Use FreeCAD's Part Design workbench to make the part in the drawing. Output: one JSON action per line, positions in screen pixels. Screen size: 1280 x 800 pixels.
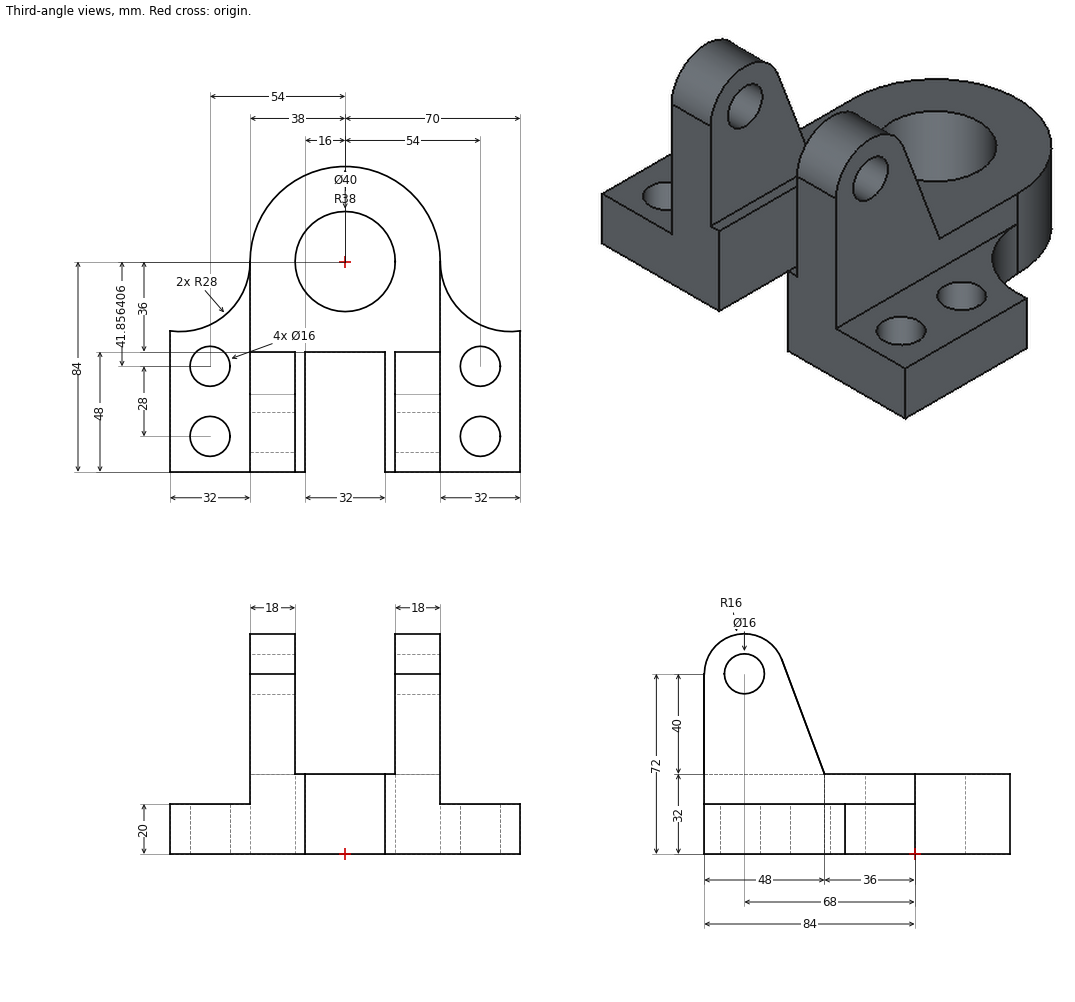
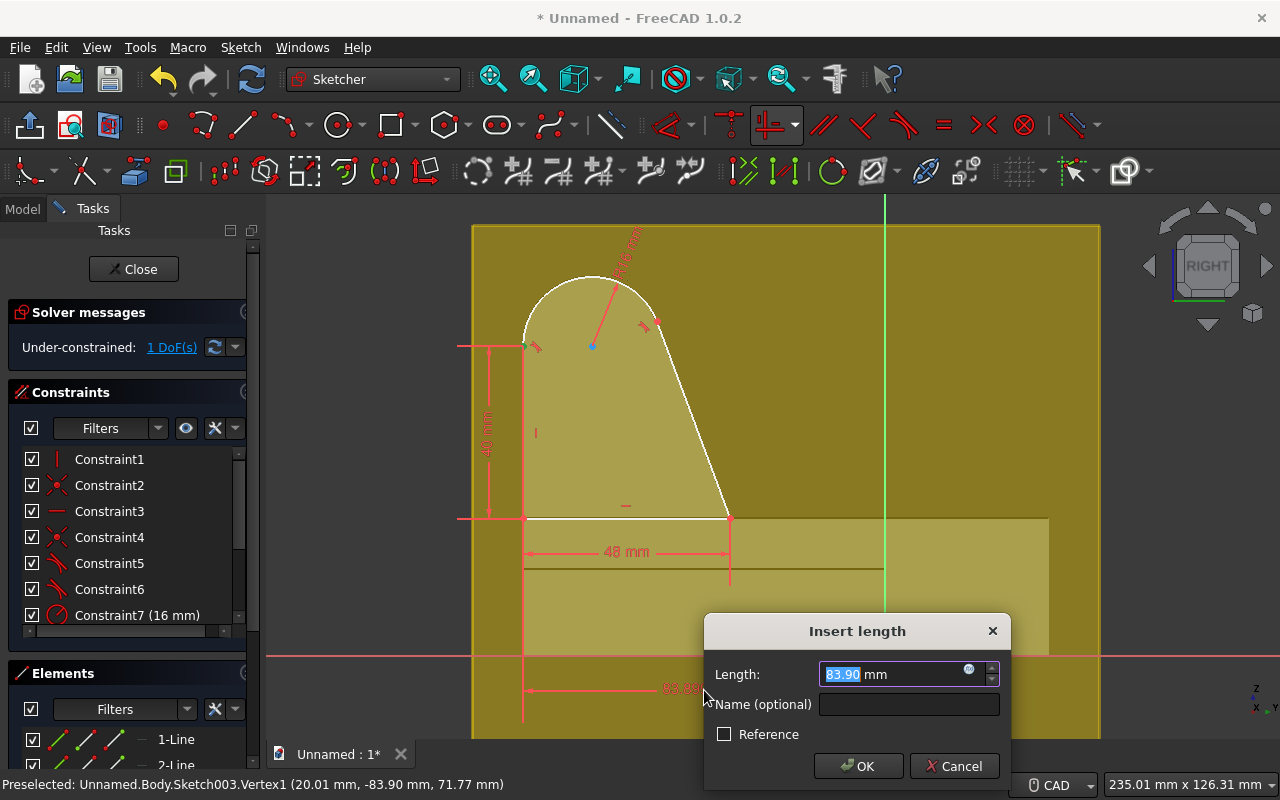
{"action": "type", "text": "84"}
{"action": "key", "text": "Return"}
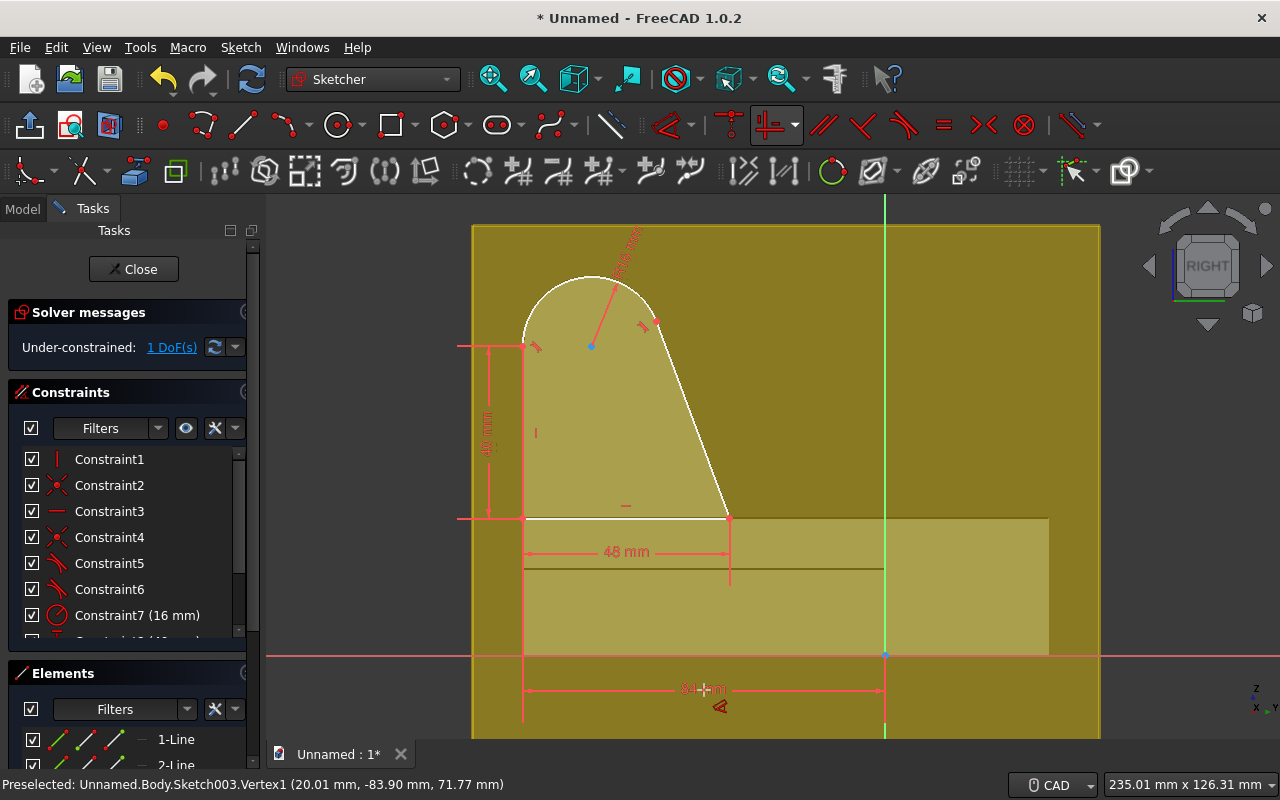
{"action": "left_click", "coordinate": [523, 346]}
{"action": "left_click", "coordinate": [919, 501]}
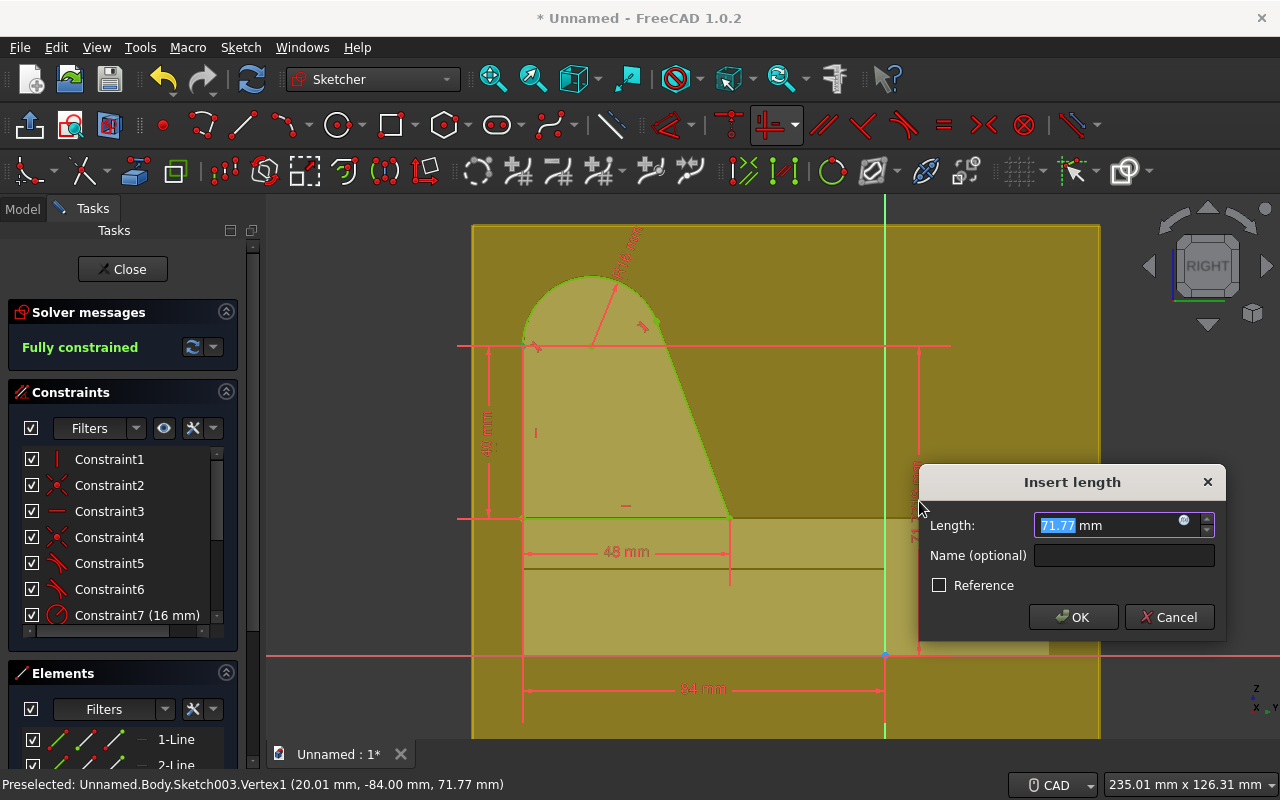
{"action": "type", "text": "72"}
{"action": "key", "text": "Return"}
{"action": "key", "text": "Escape"}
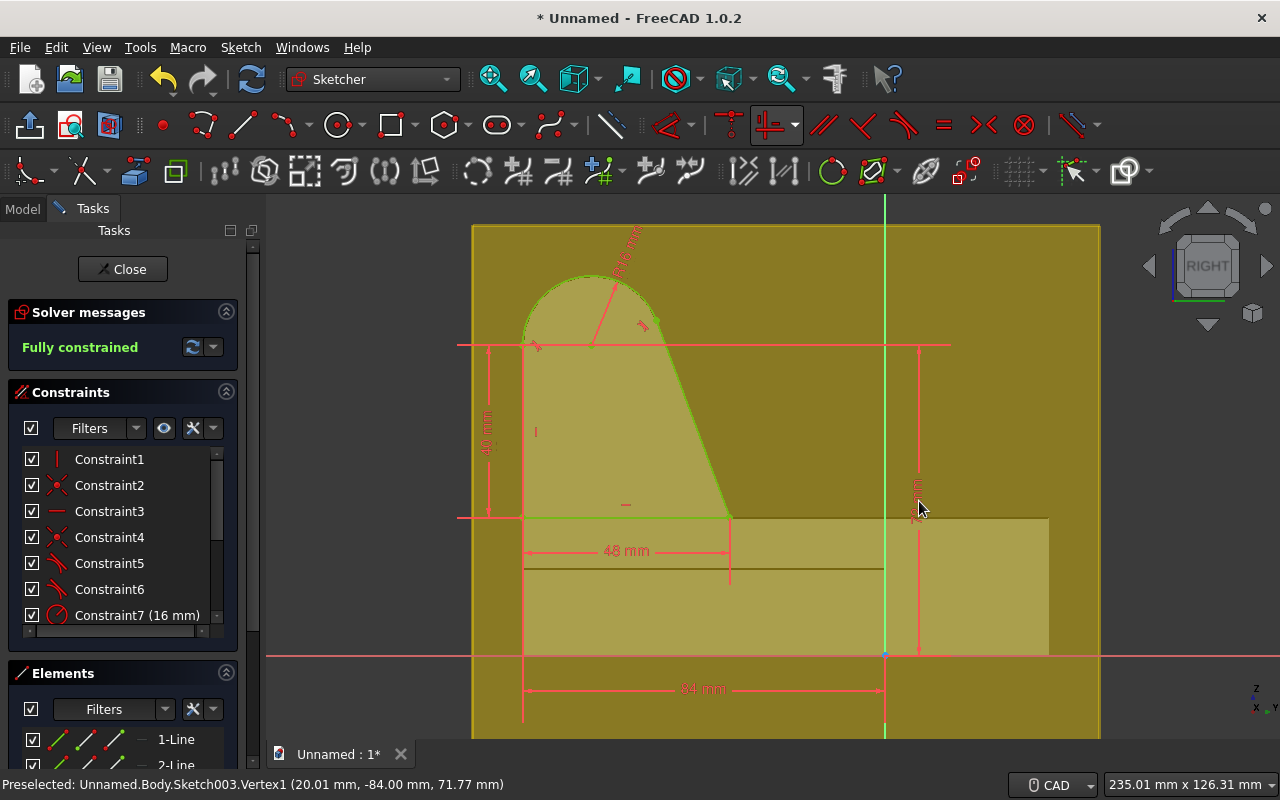
{"action": "left_click", "coordinate": [123, 269]}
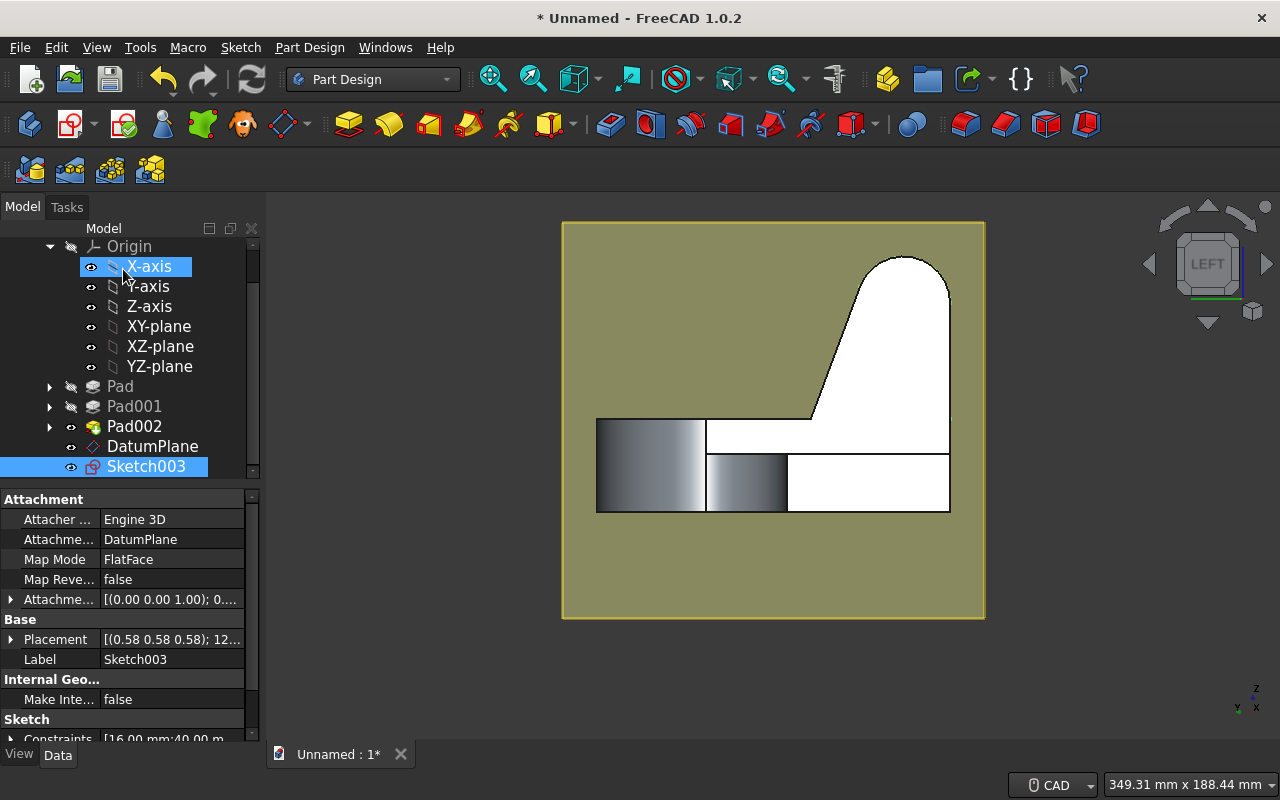
{"action": "left_click", "coordinate": [350, 124]}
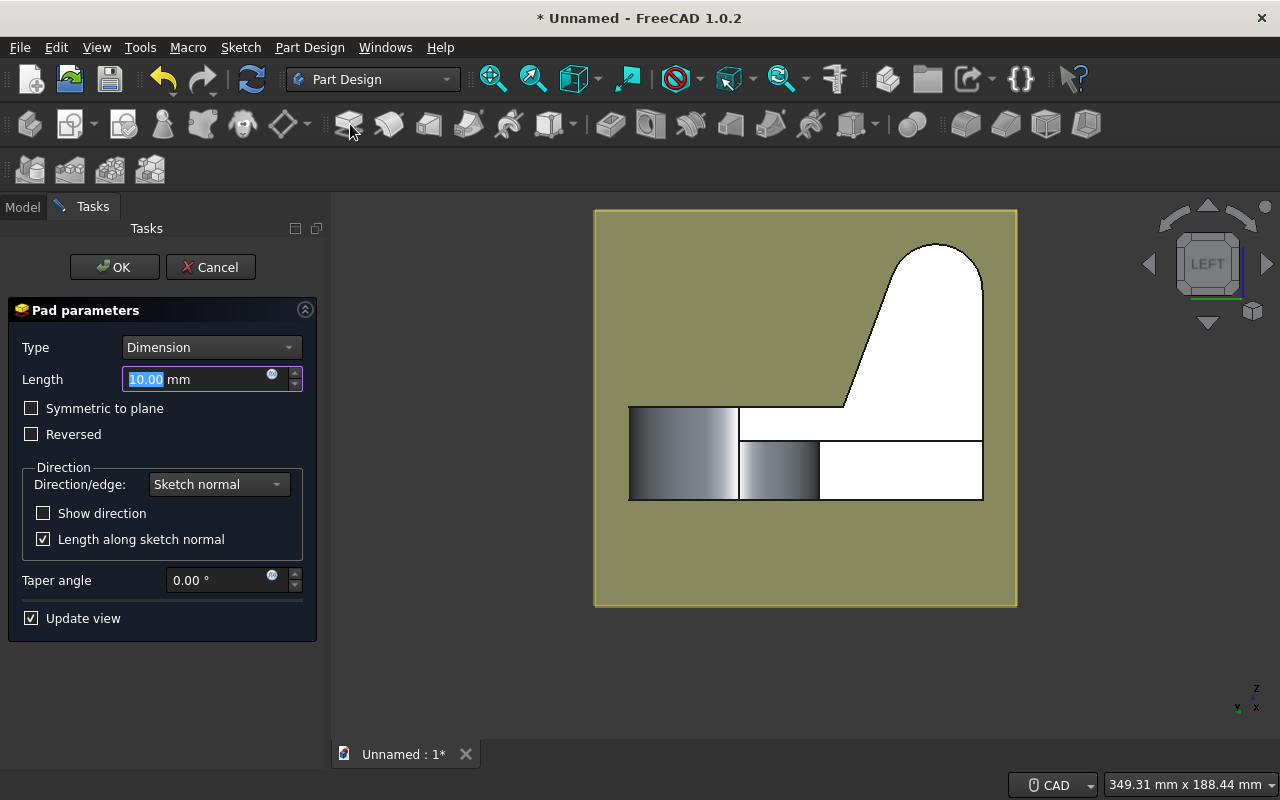
{"action": "type", "text": "18"}
{"action": "key", "text": "Tab"}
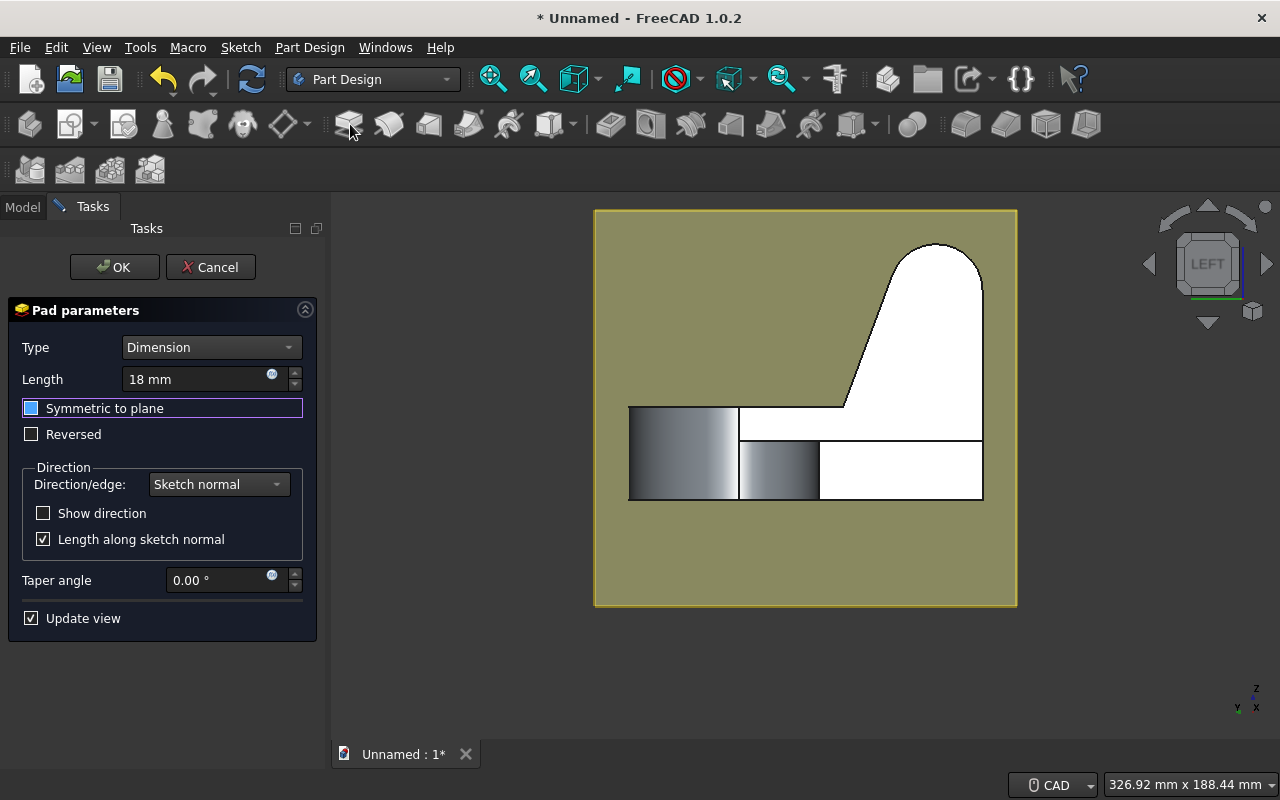
{"action": "left_click", "coordinate": [115, 267]}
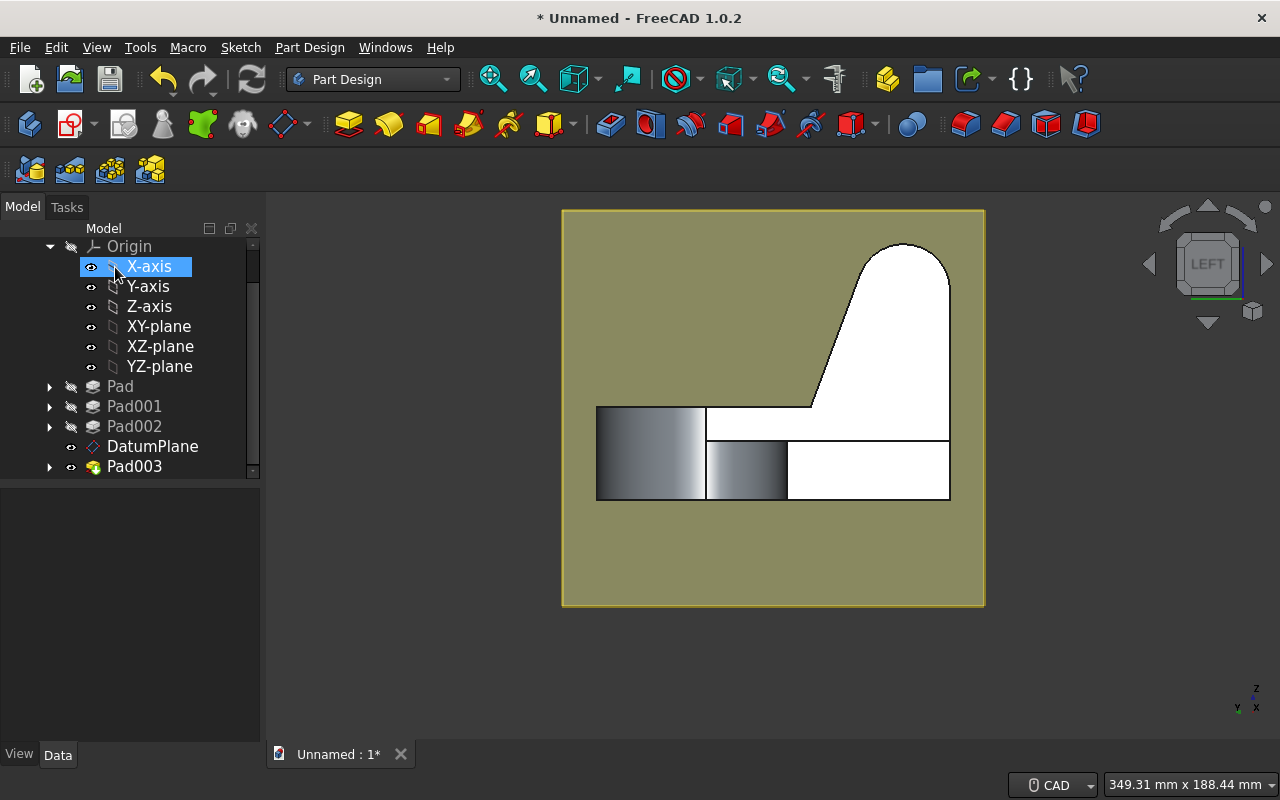
{"action": "left_click", "coordinate": [116, 447]}
{"action": "key", "text": "space"}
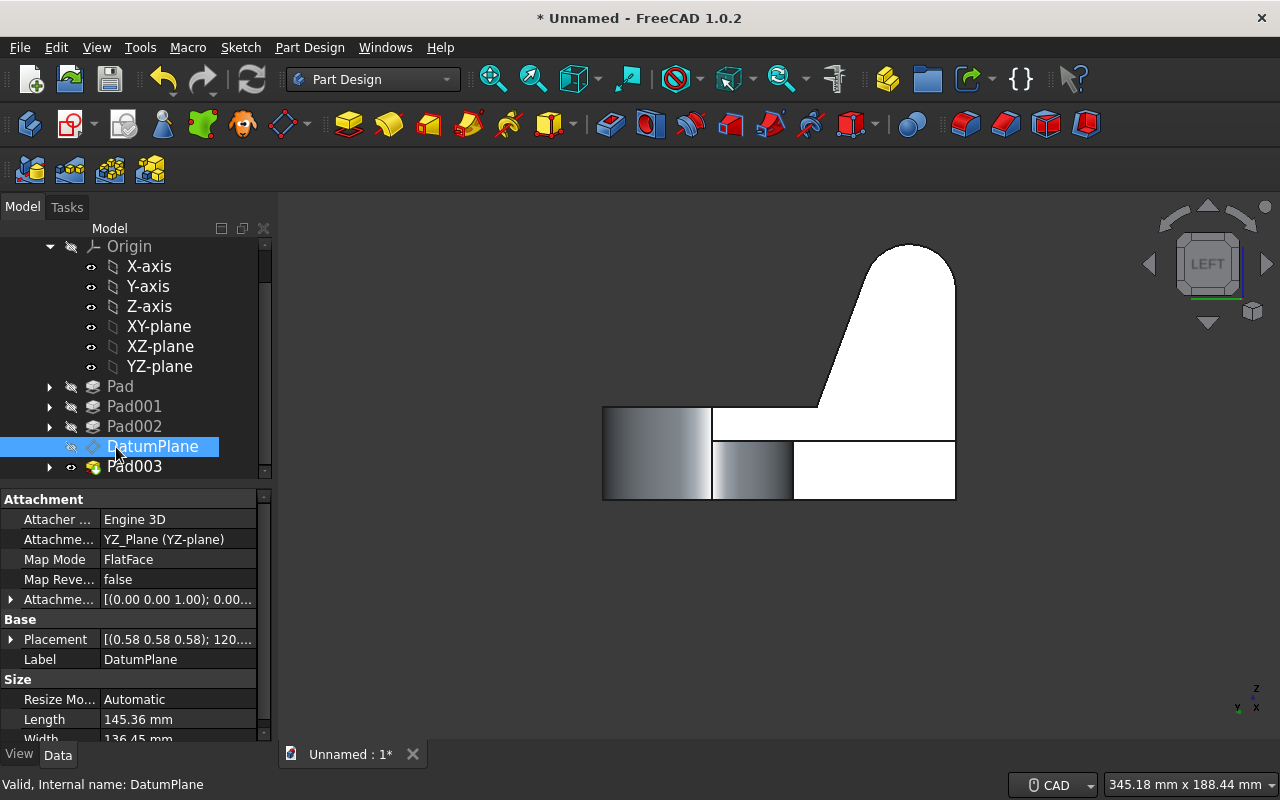
{"action": "key", "text": "0"}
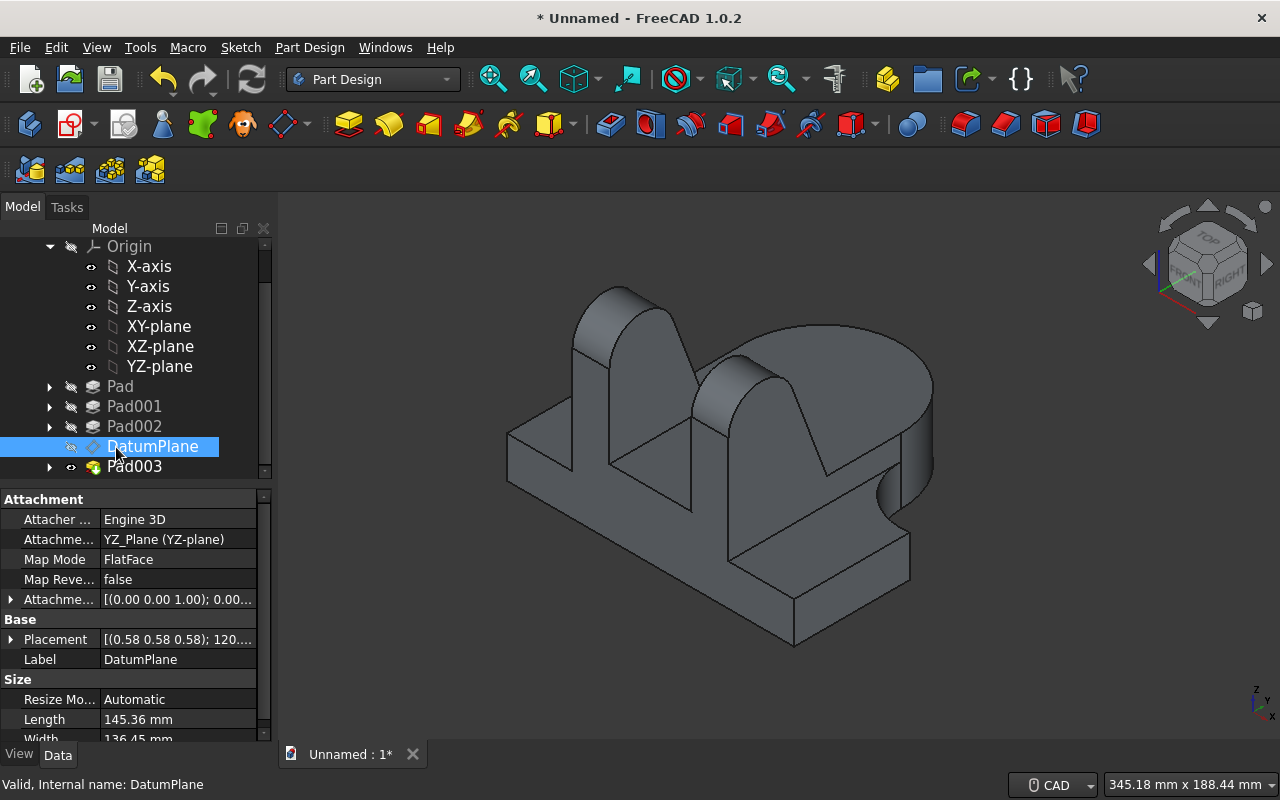
{"action": "left_click", "coordinate": [494, 80]}